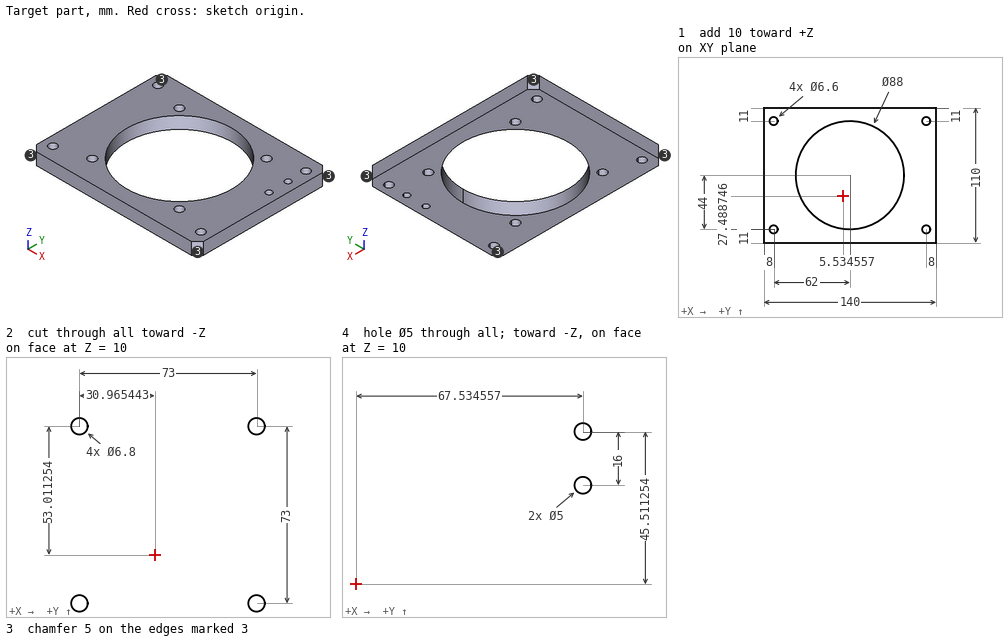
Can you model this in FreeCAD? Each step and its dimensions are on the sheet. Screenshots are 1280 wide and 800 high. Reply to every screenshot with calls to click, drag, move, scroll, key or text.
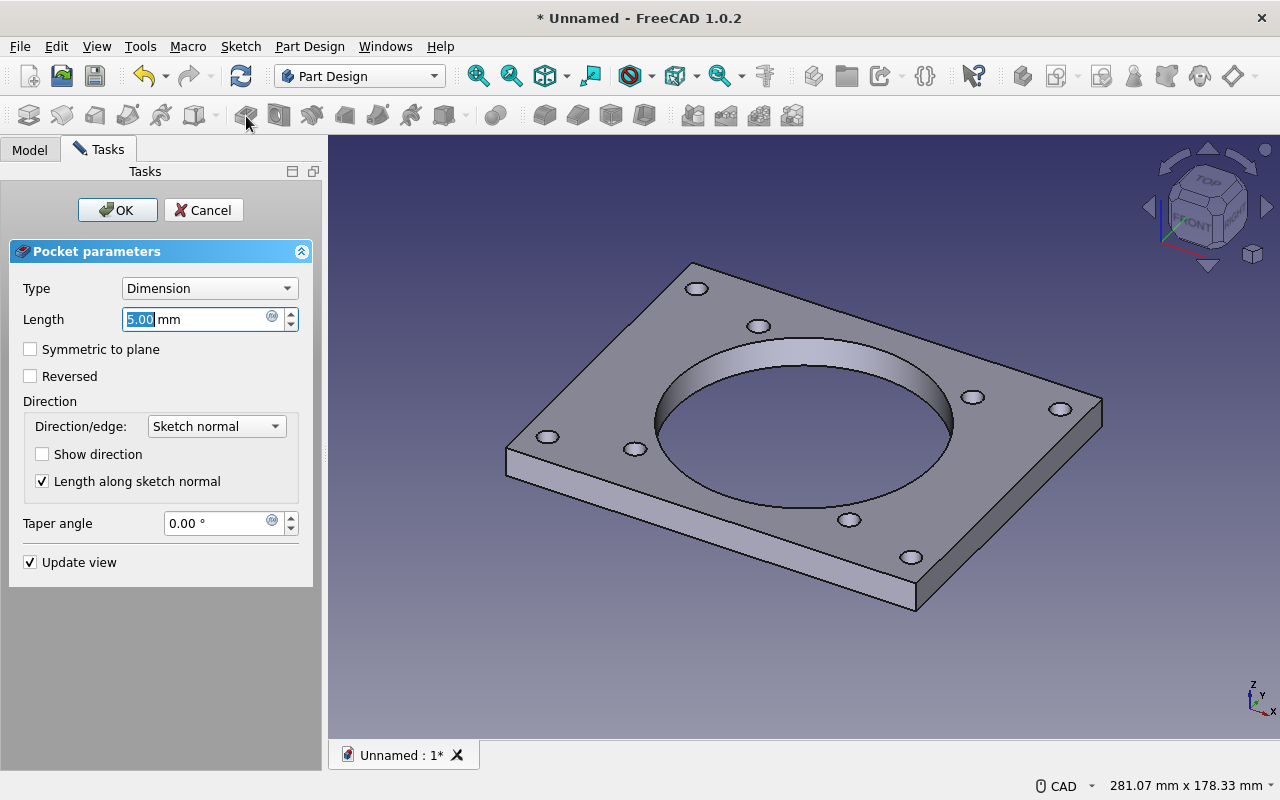
click(210, 288)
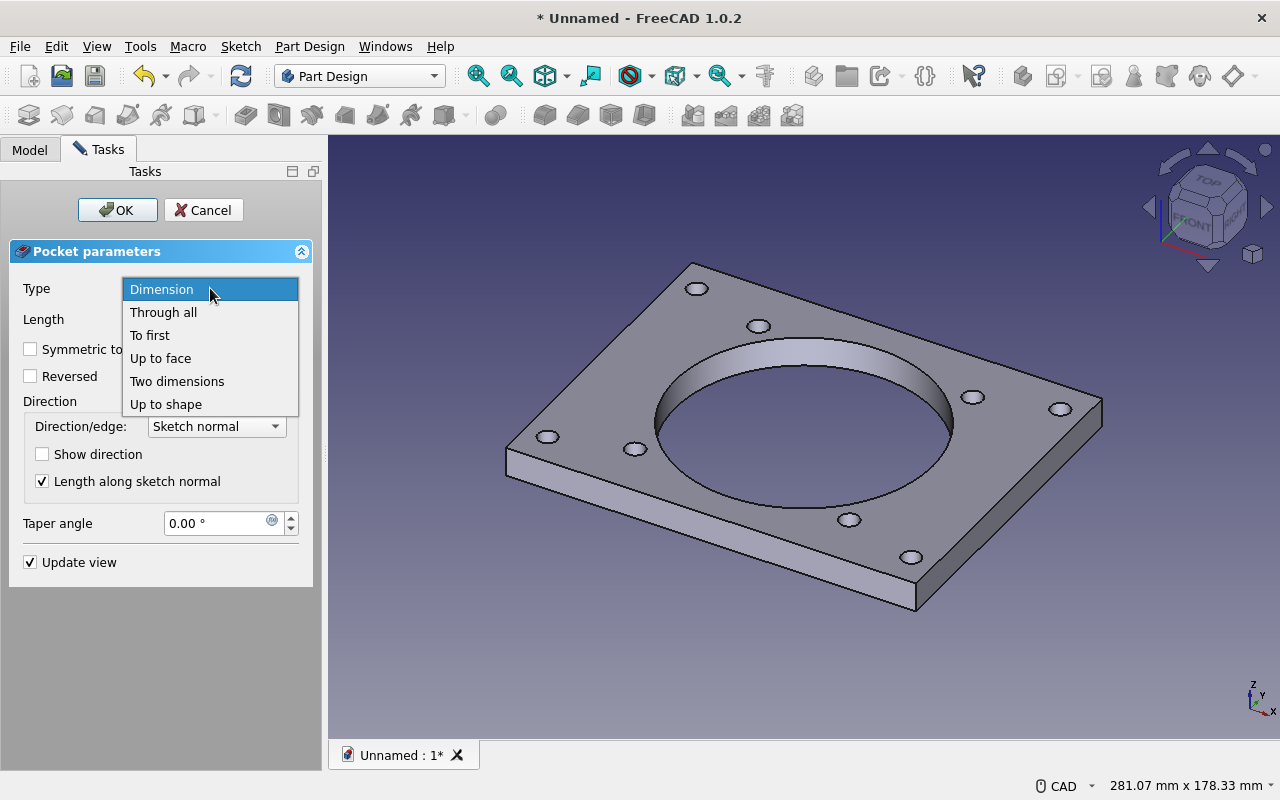
click(208, 312)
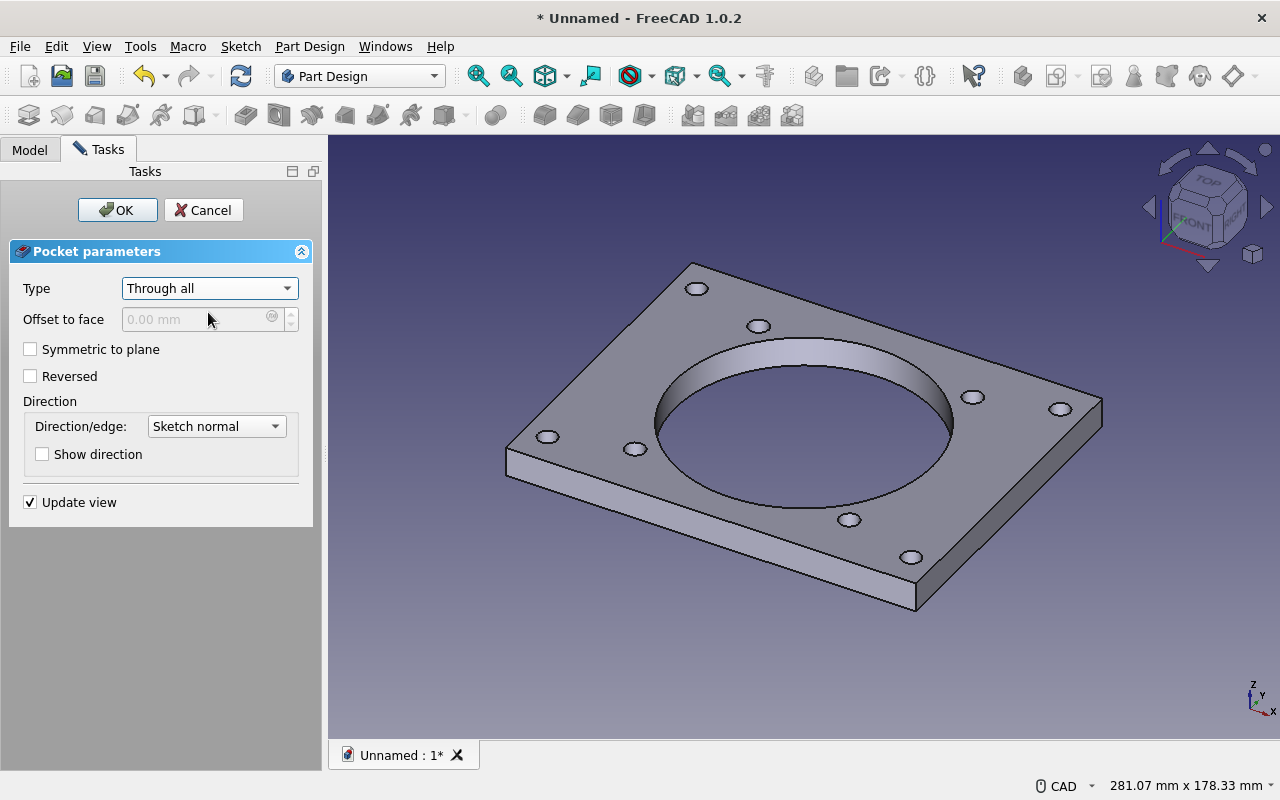
click(118, 210)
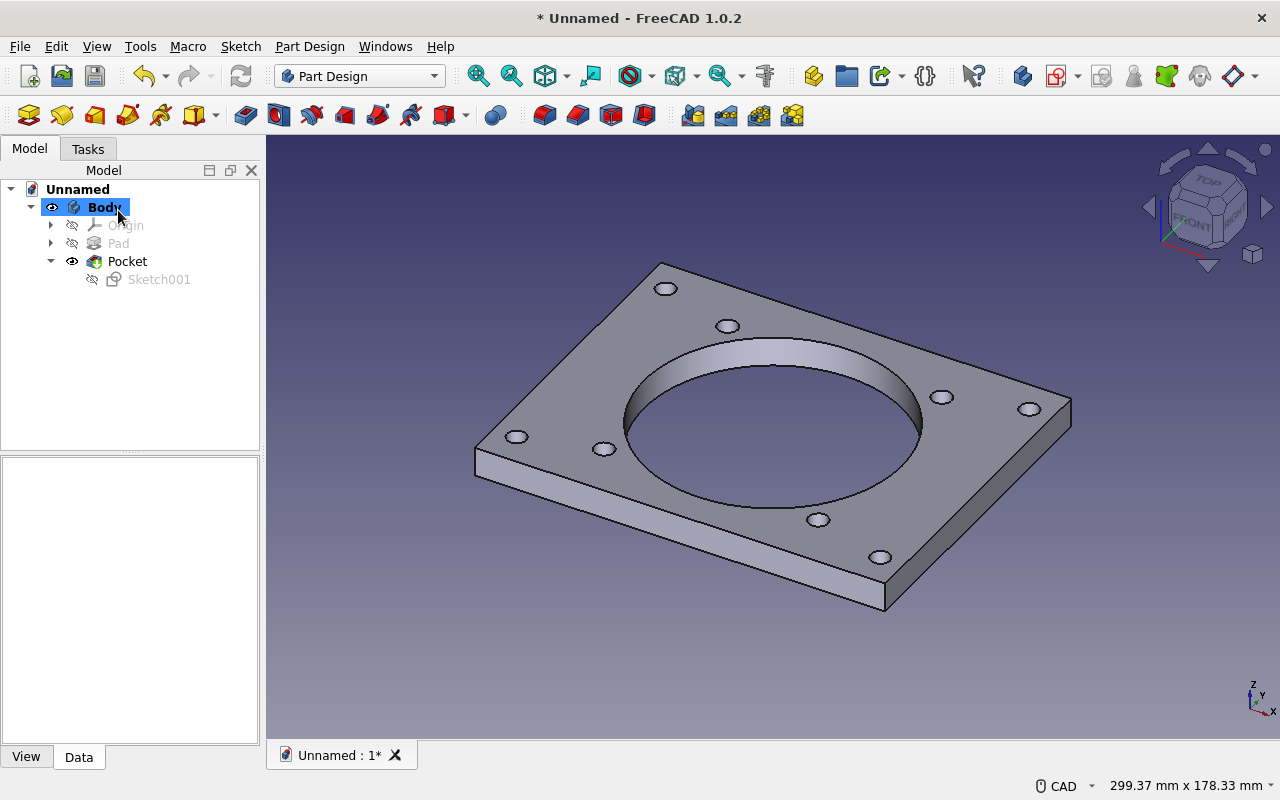
click(885, 597)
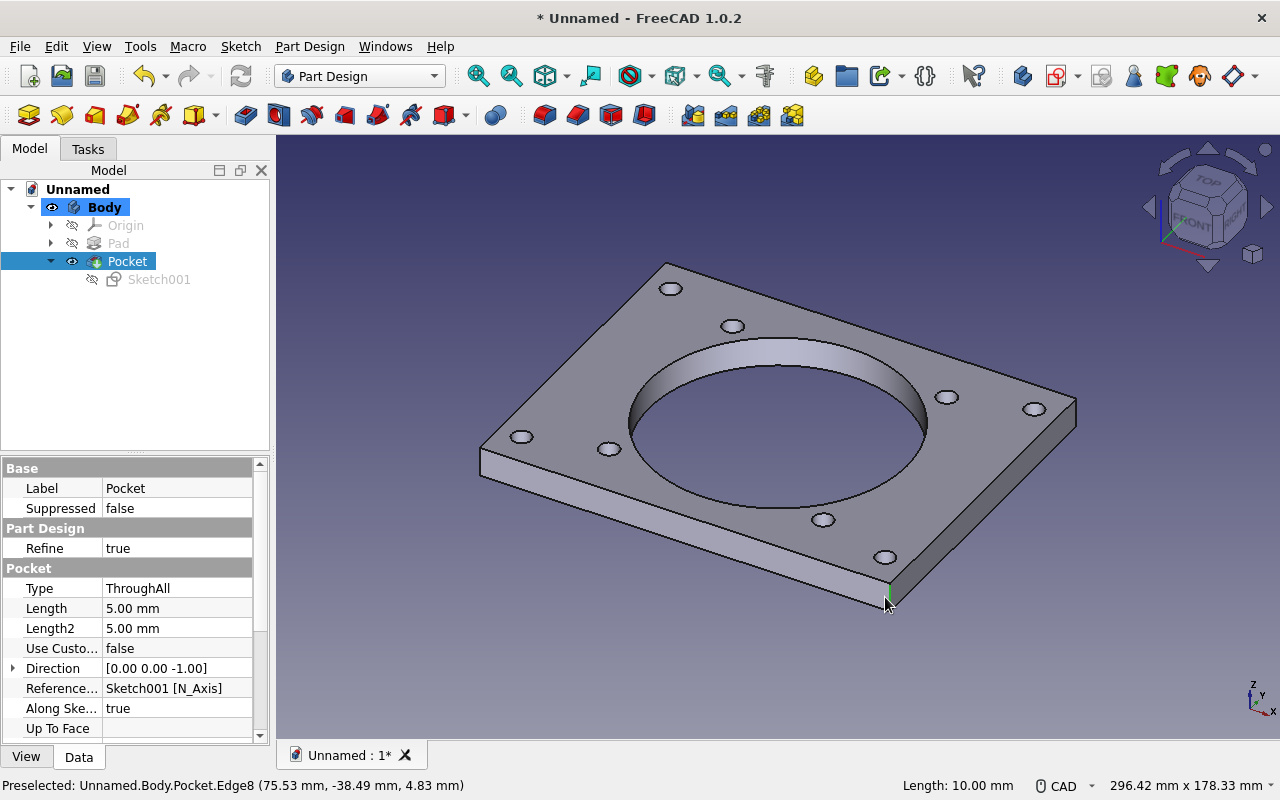
key(0)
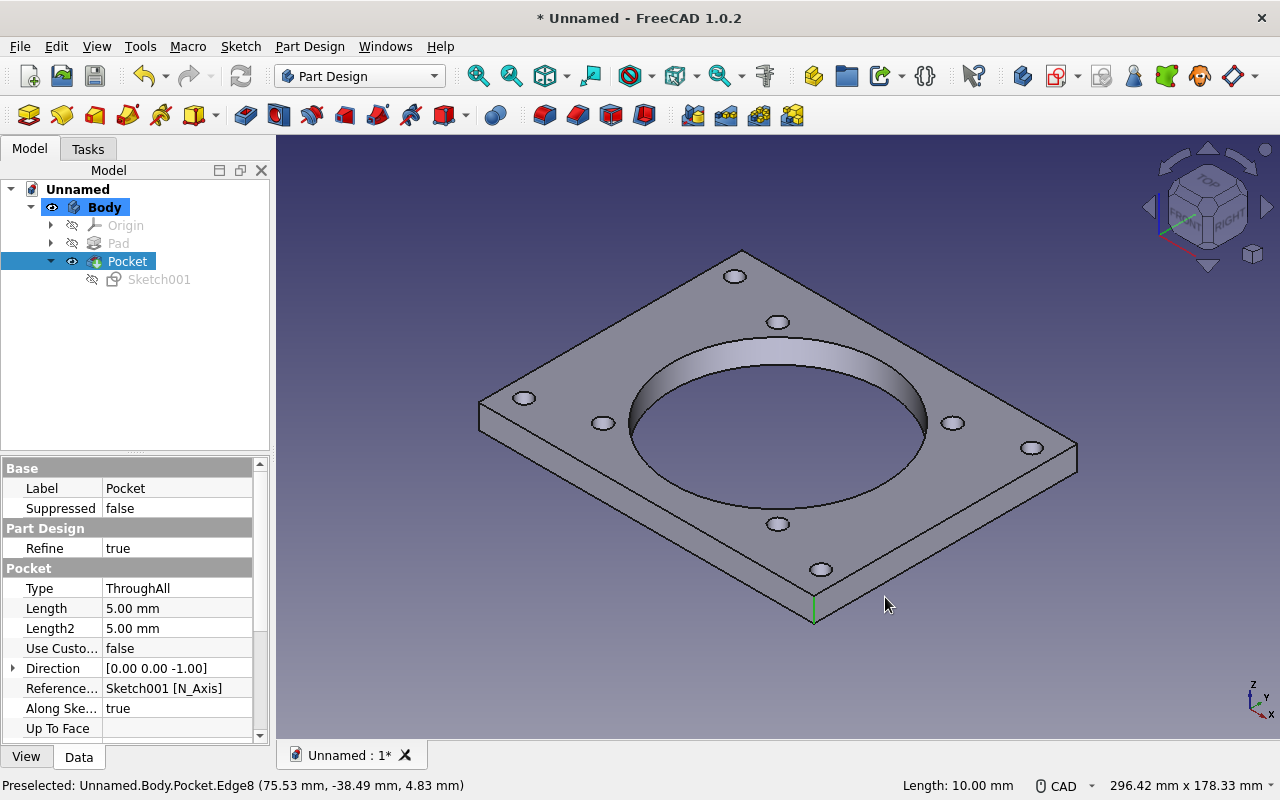
key(2)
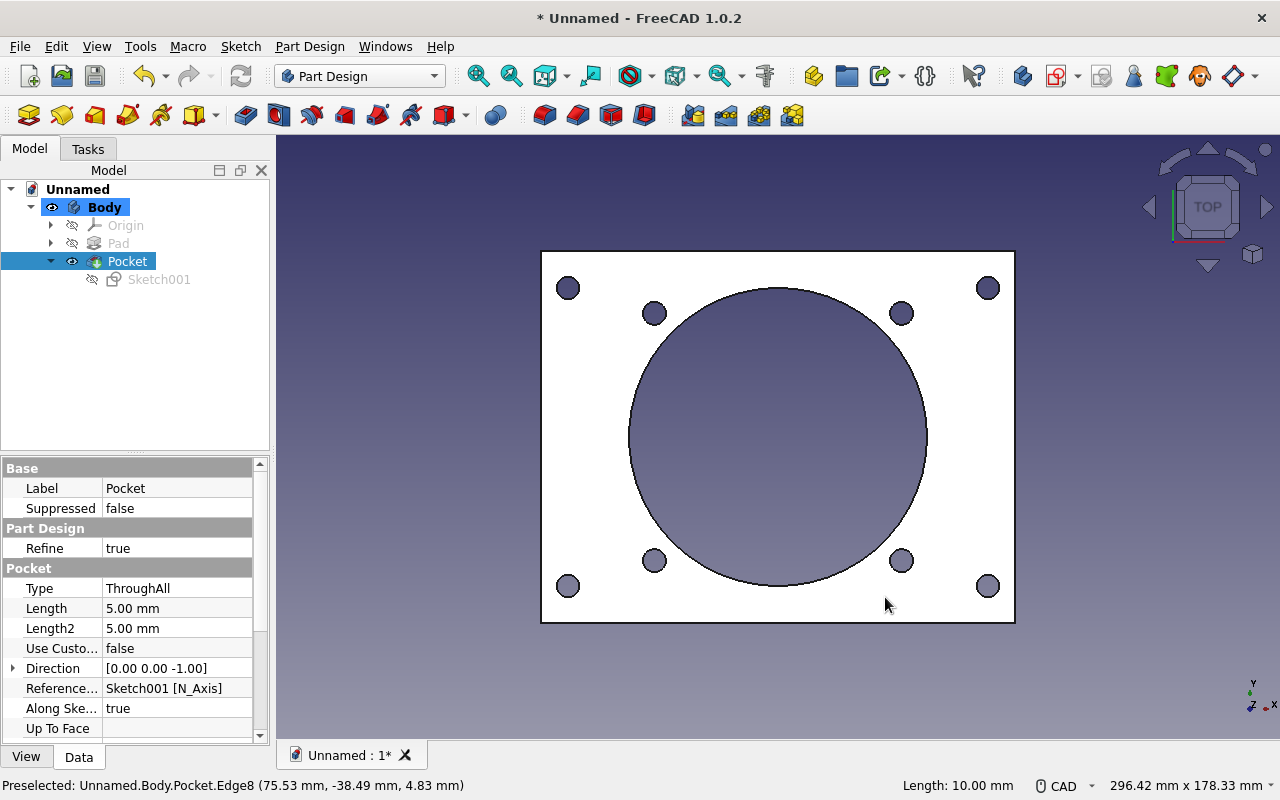
key(1)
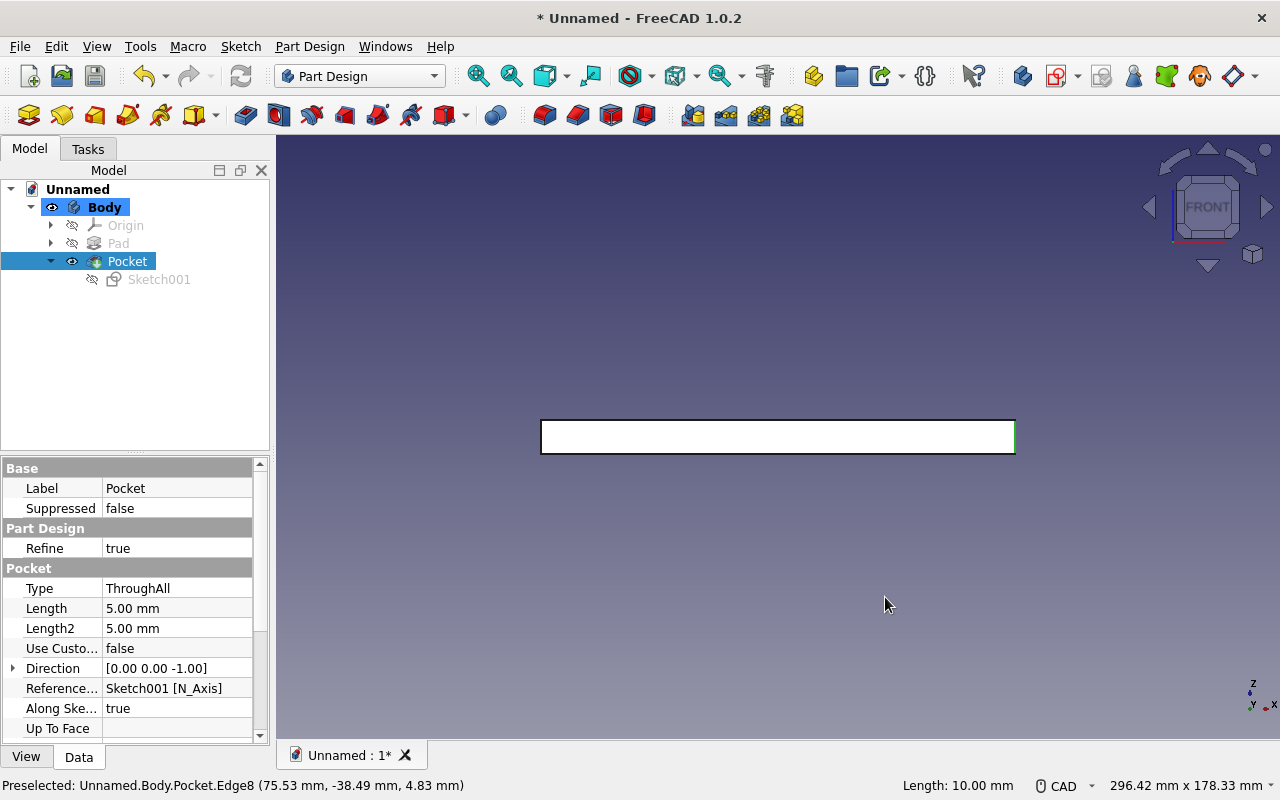
click(541, 436, ctrl)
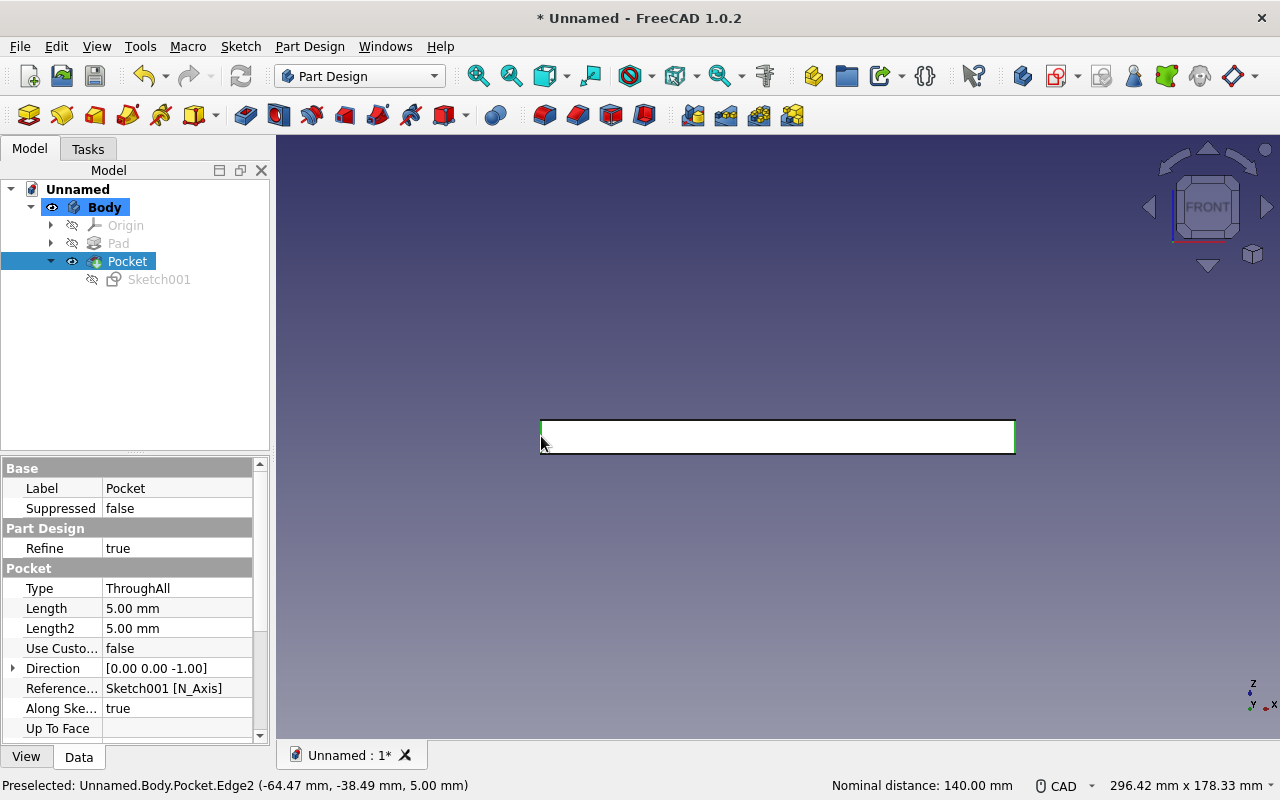
key(3)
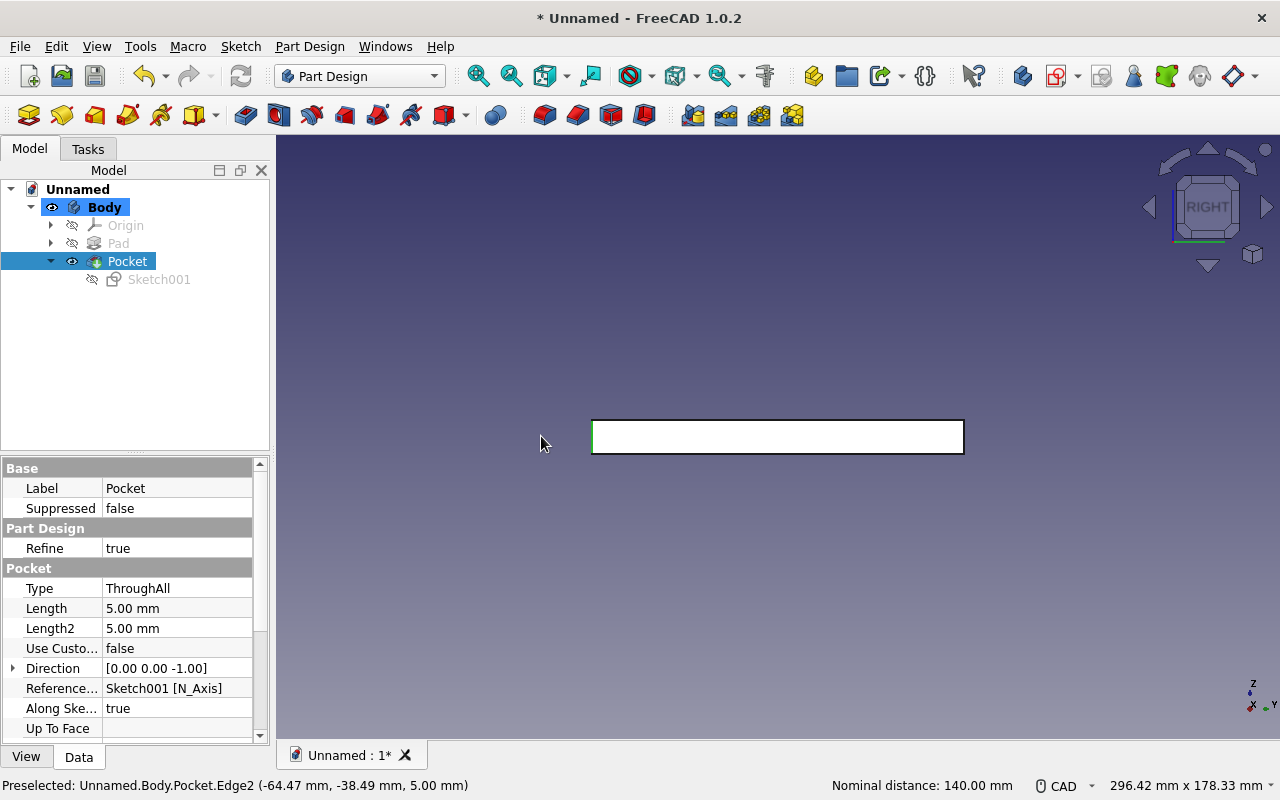
click(479, 76)